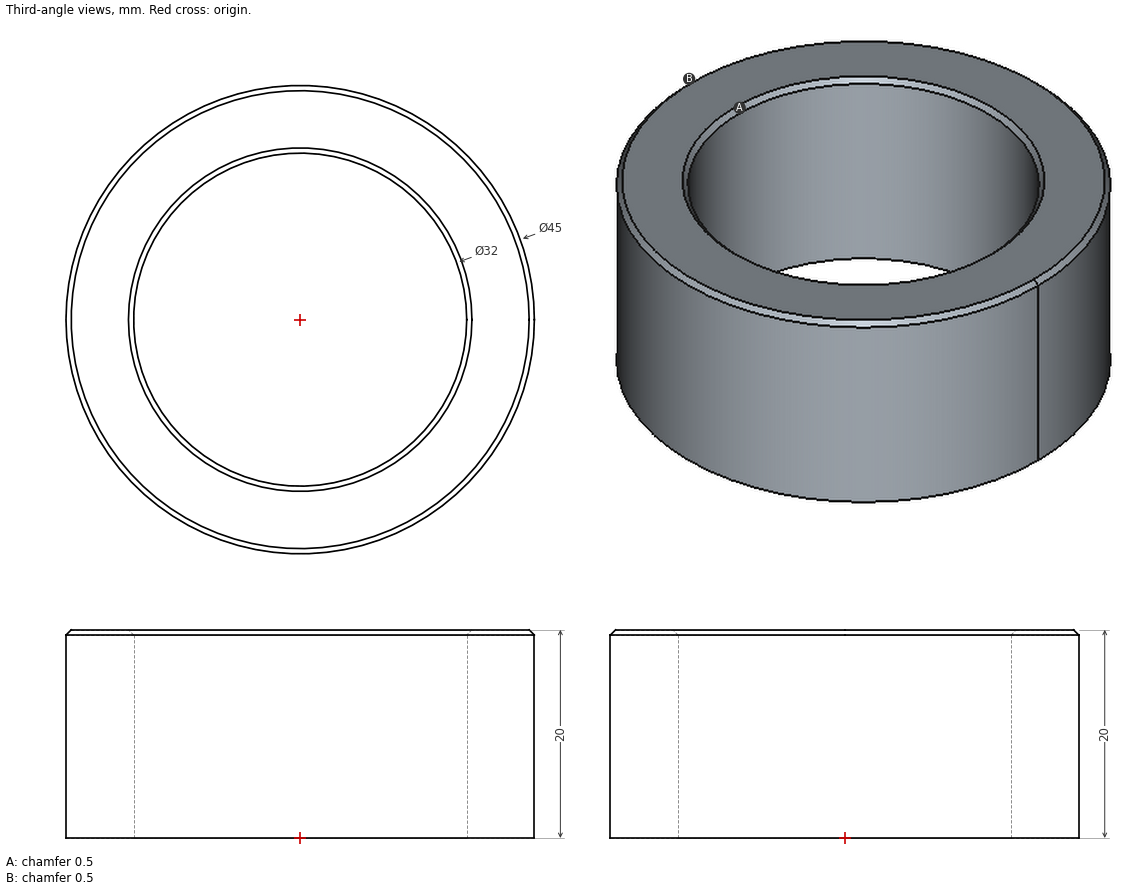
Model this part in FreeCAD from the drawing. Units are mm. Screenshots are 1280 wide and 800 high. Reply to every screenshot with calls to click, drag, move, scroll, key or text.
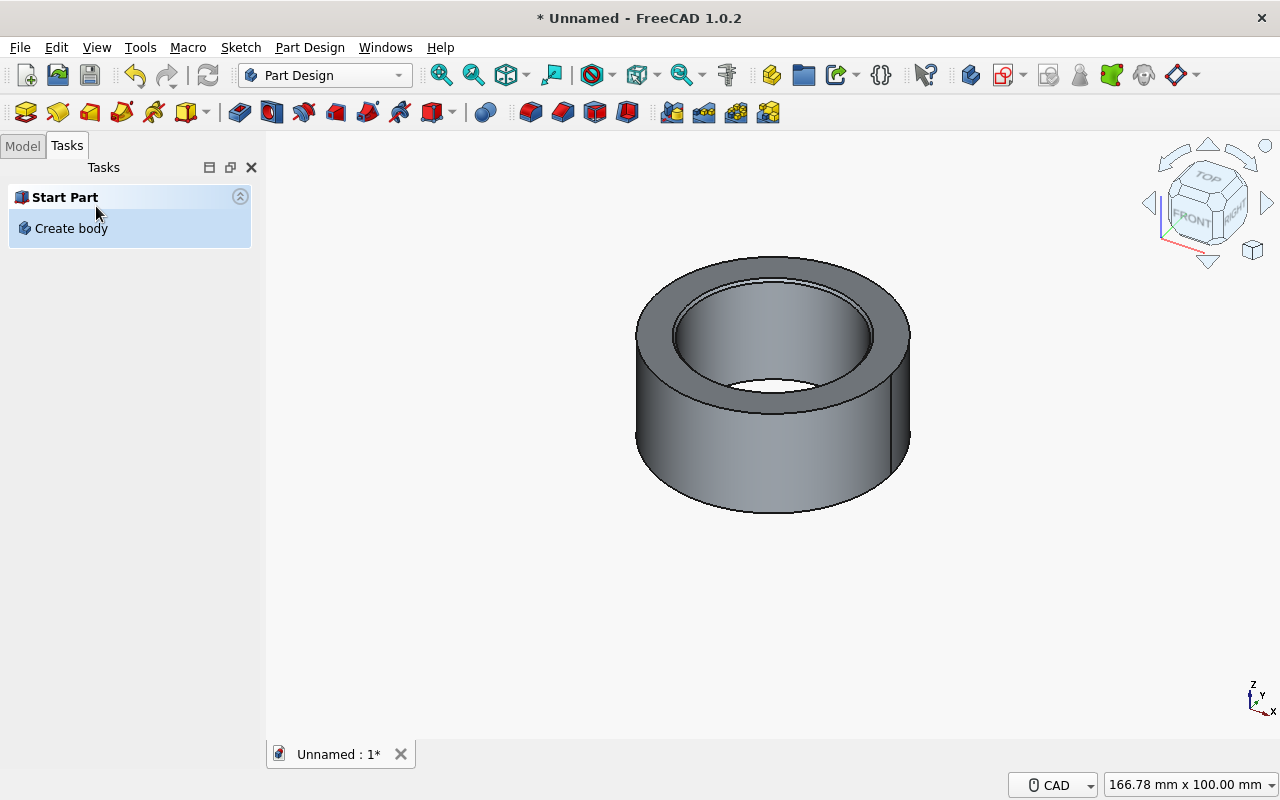
click(637, 343)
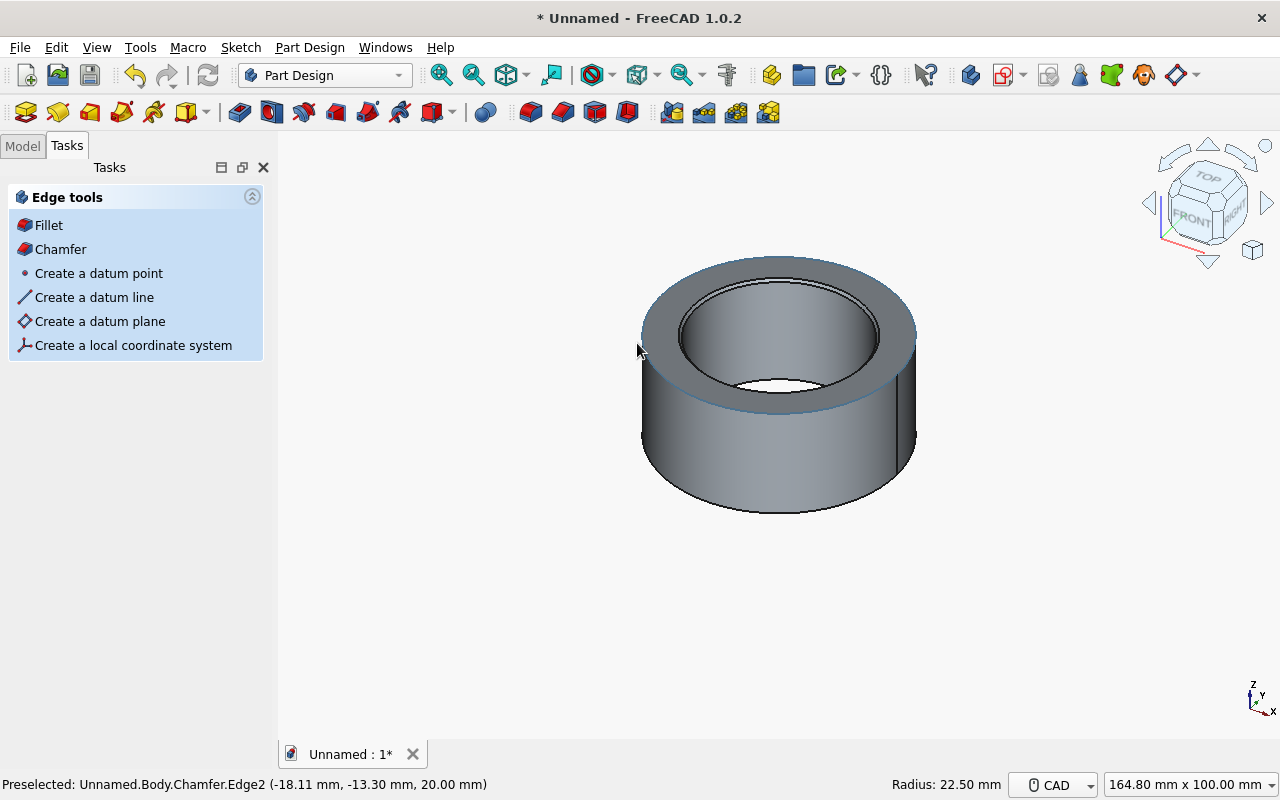
click(564, 112)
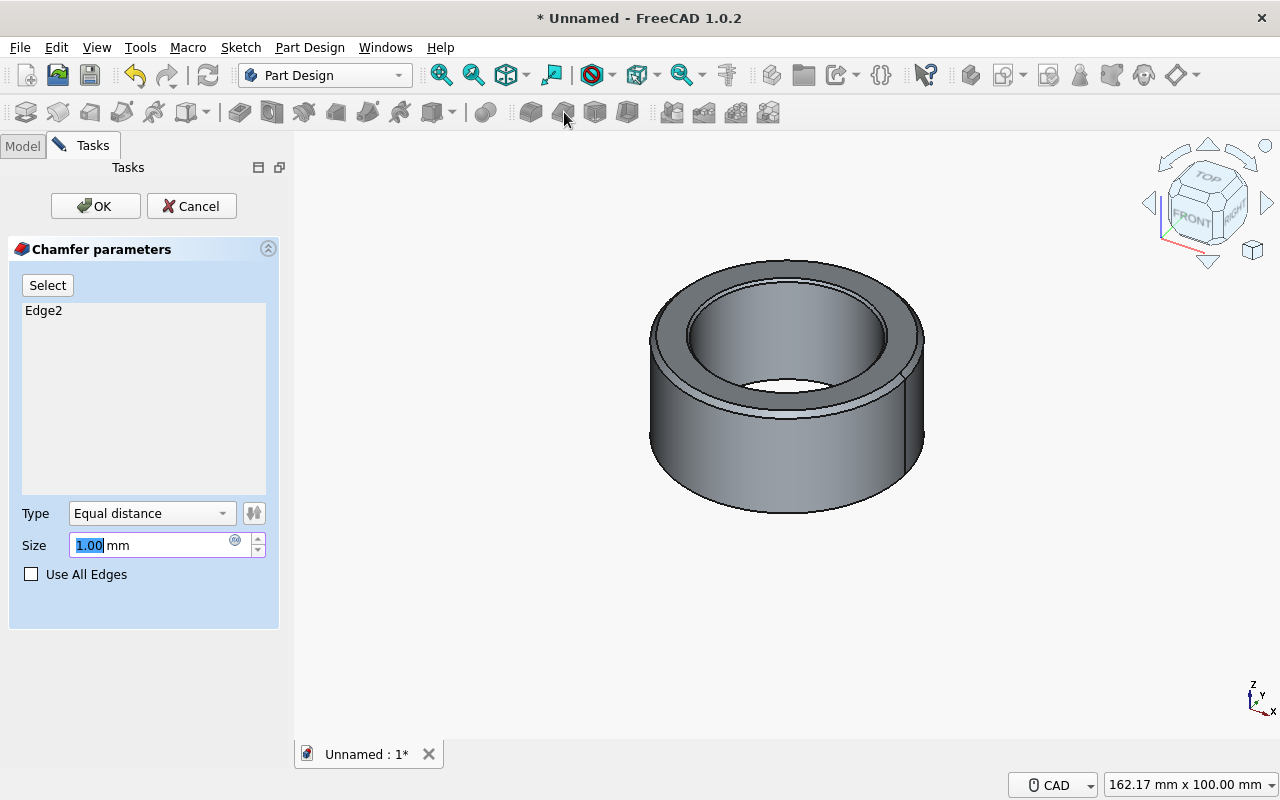
text(0.5)
key(Tab)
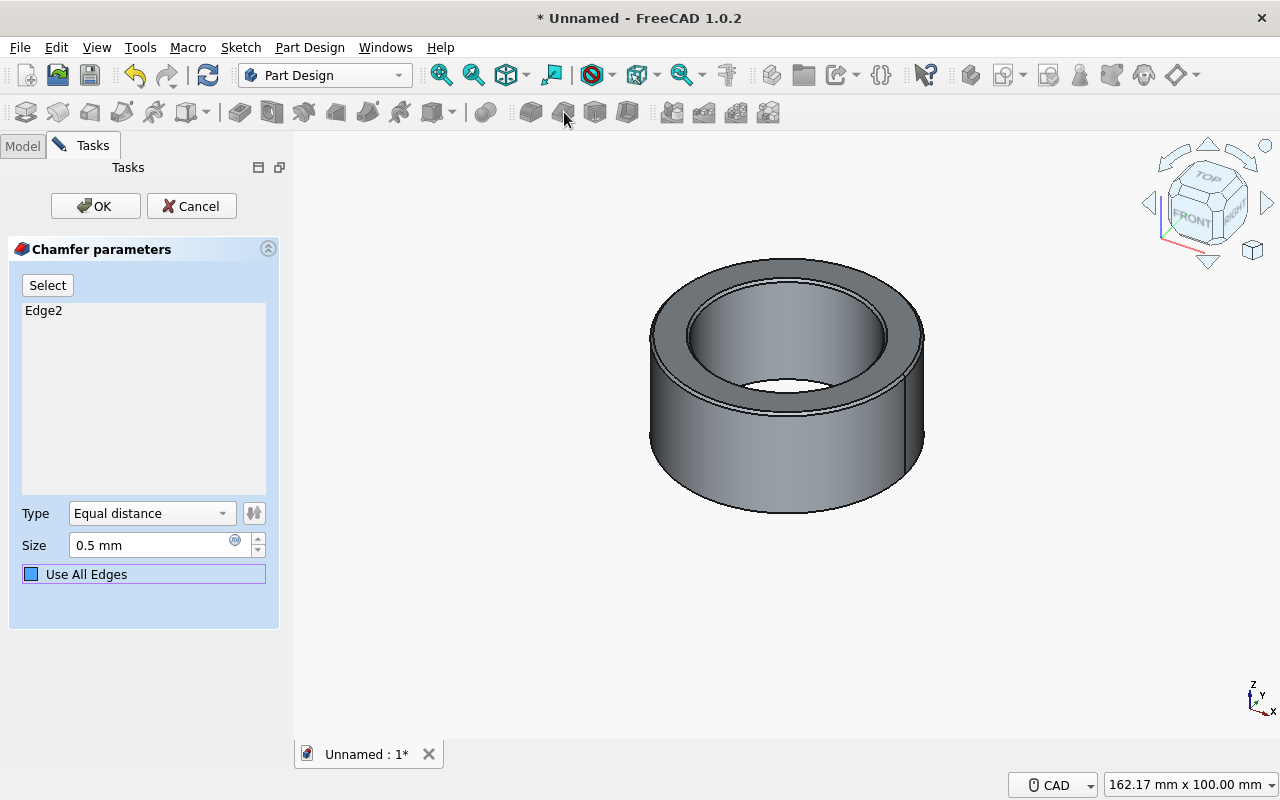
click(96, 206)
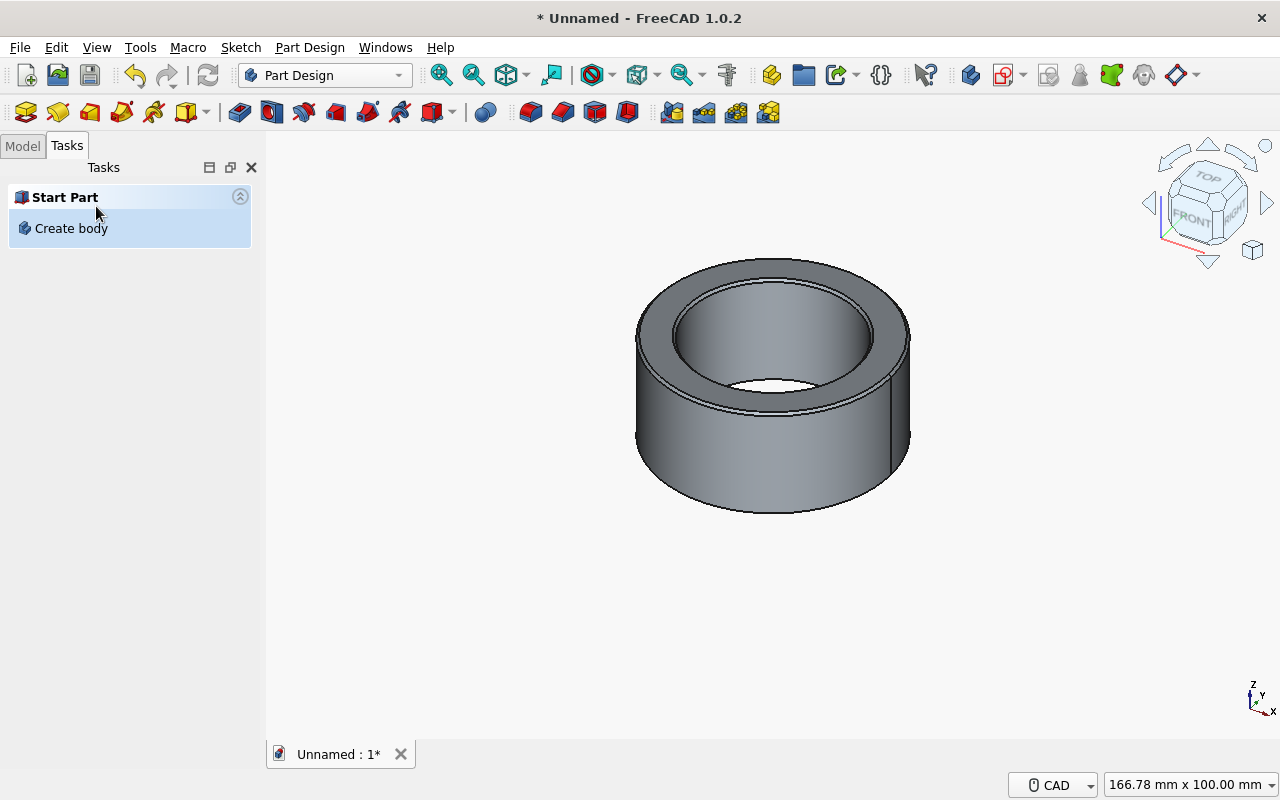
key(0)